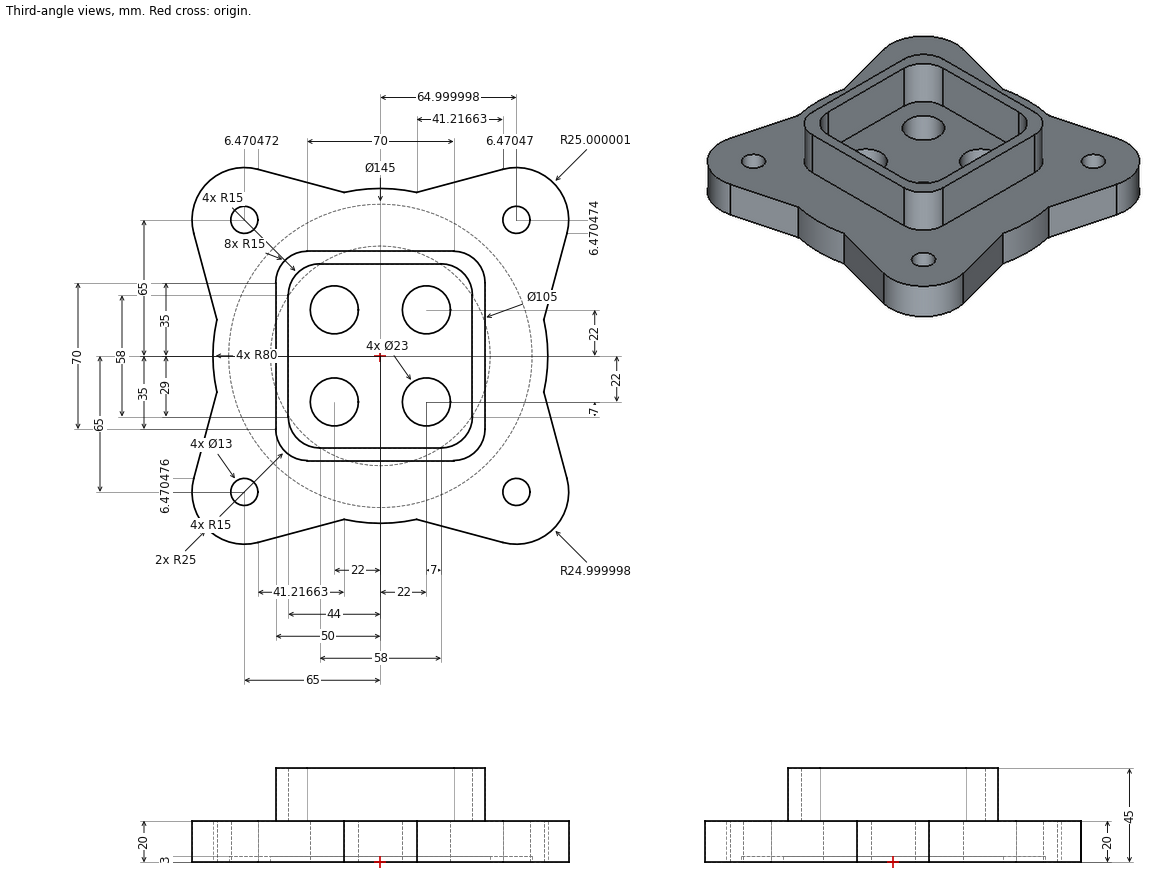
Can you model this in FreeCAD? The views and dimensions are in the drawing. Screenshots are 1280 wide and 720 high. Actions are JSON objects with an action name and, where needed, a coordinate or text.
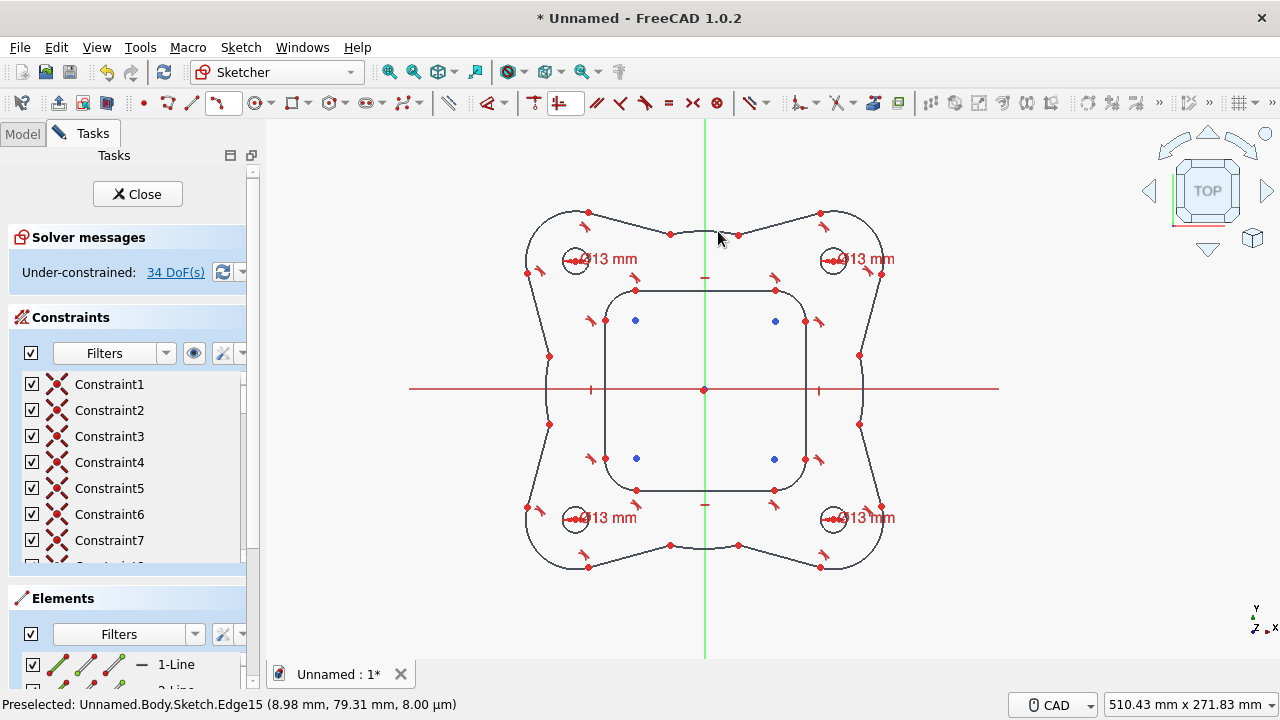
{"action": "scroll", "coordinate": [704, 390], "scroll_direction": "up", "scroll_amount": 6}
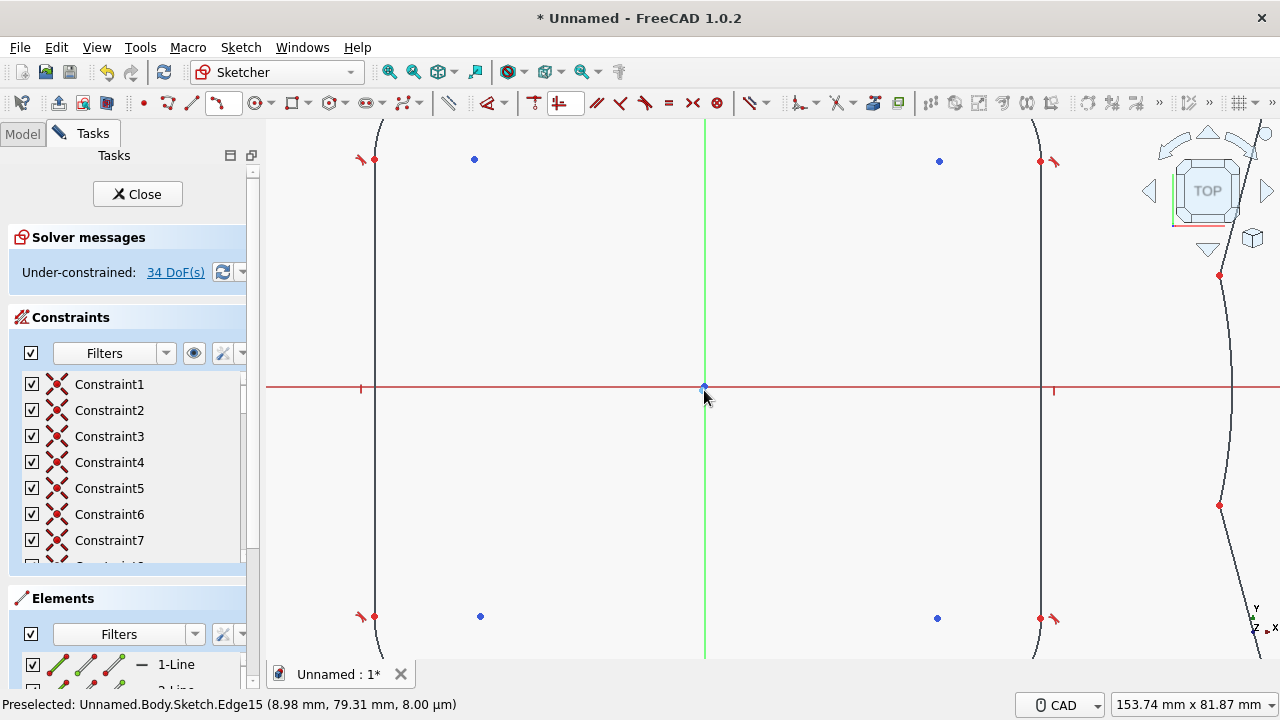
{"action": "left_click_drag", "start_coordinate": [692, 377], "coordinate": [715, 400]}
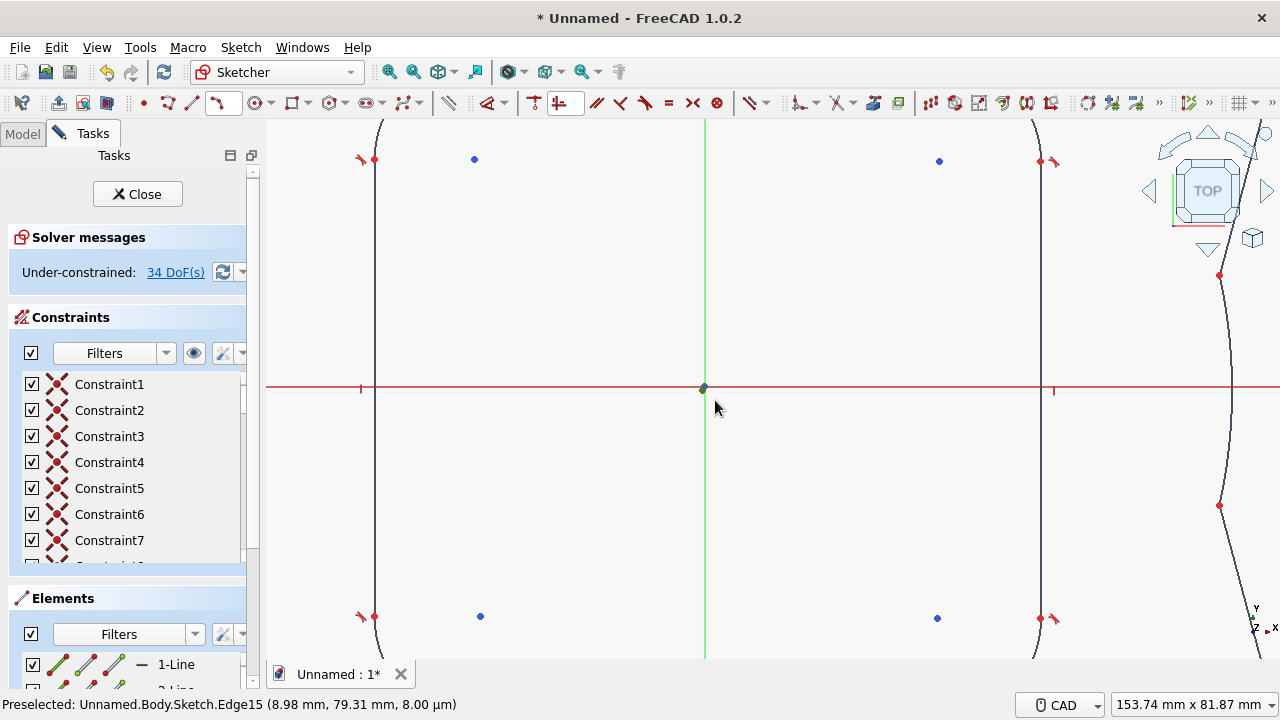
{"action": "left_click", "coordinate": [534, 104]}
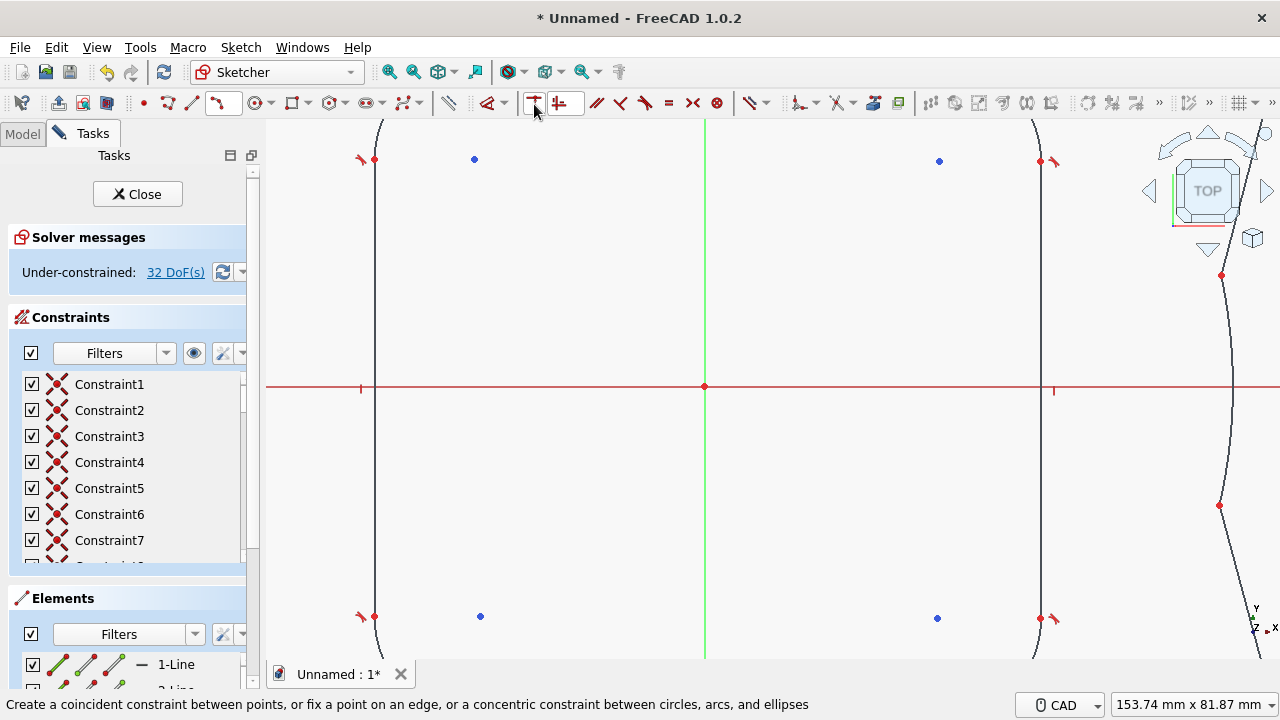
{"action": "scroll", "coordinate": [704, 390], "scroll_direction": "down", "scroll_amount": 6}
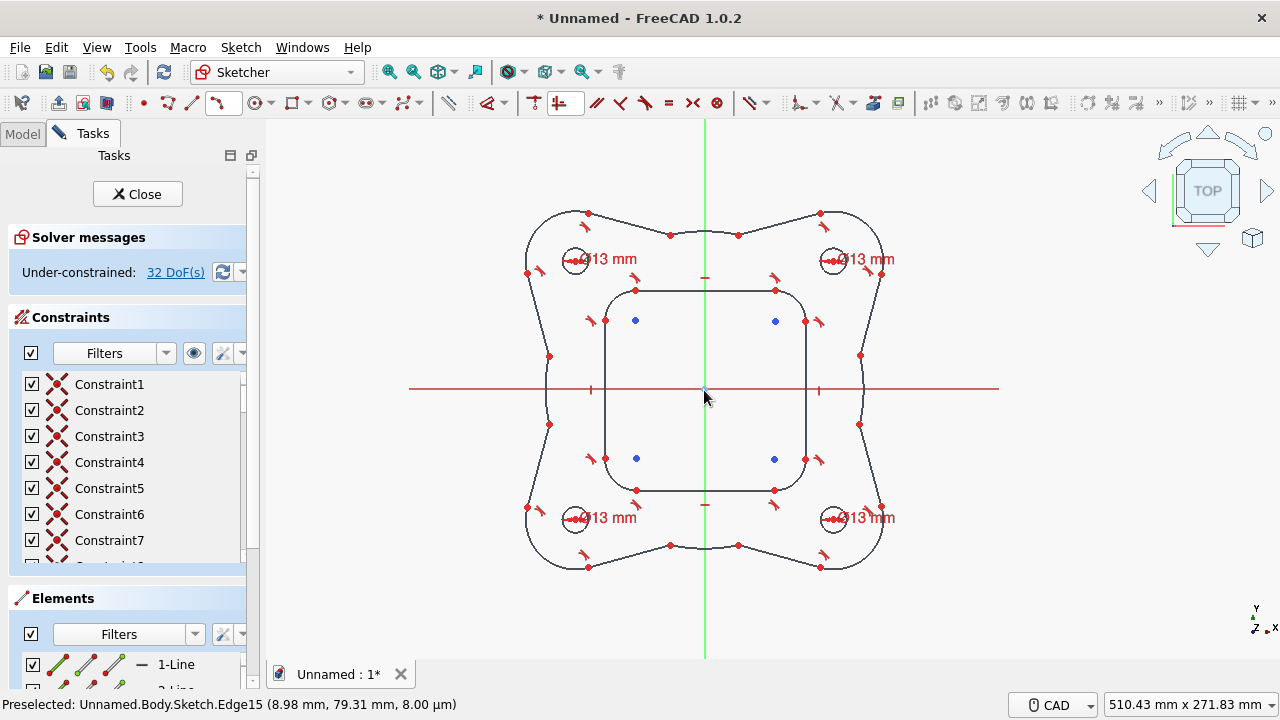
{"action": "left_click", "coordinate": [546, 377]}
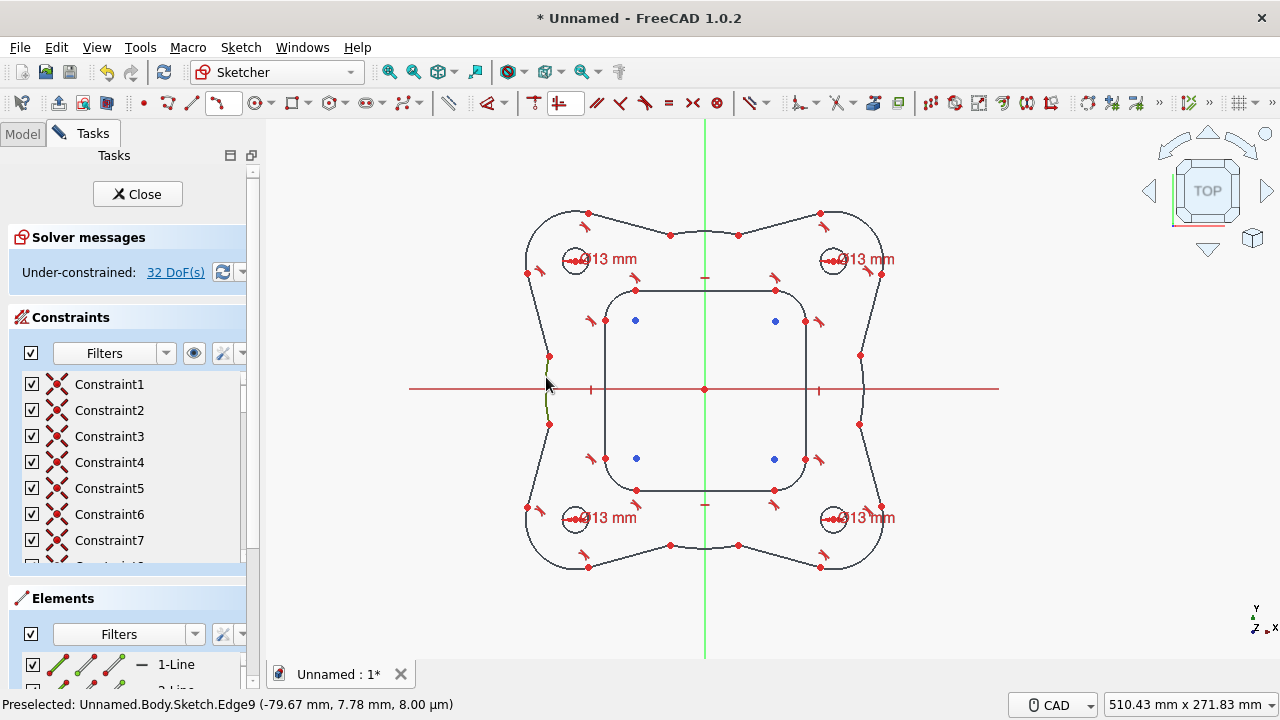
{"action": "left_click", "coordinate": [691, 548]}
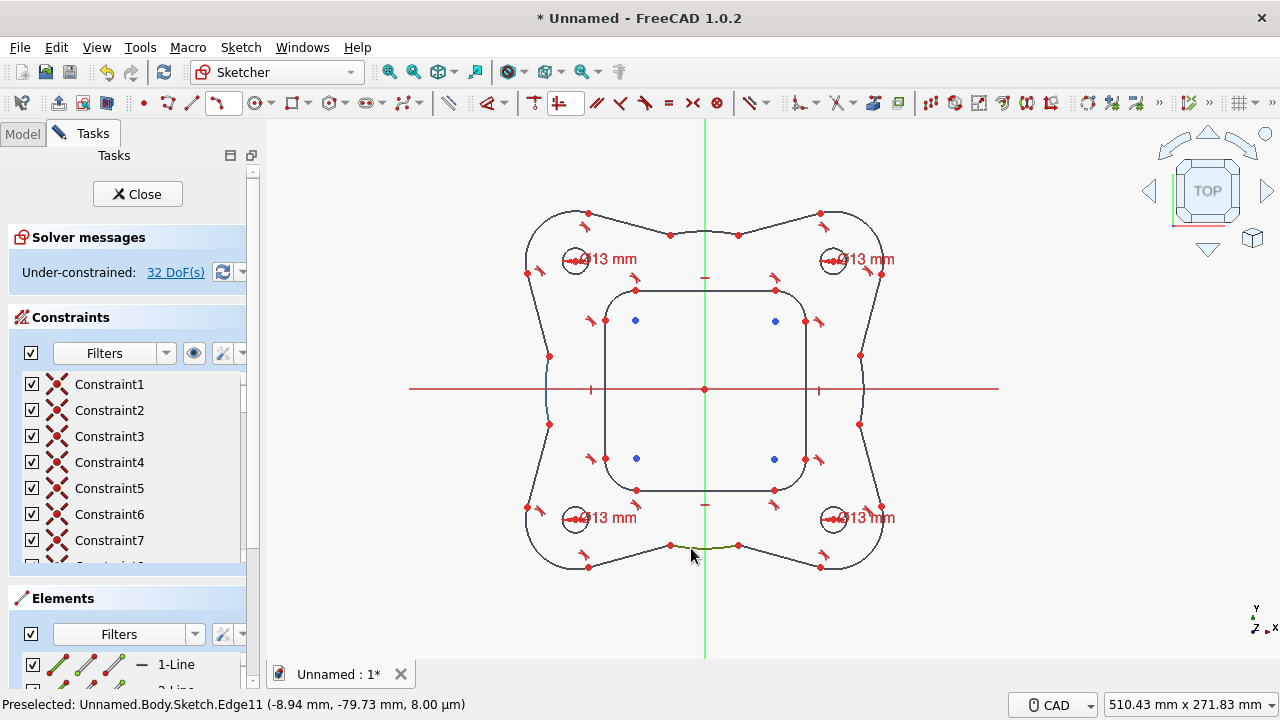
{"action": "left_click", "coordinate": [863, 404]}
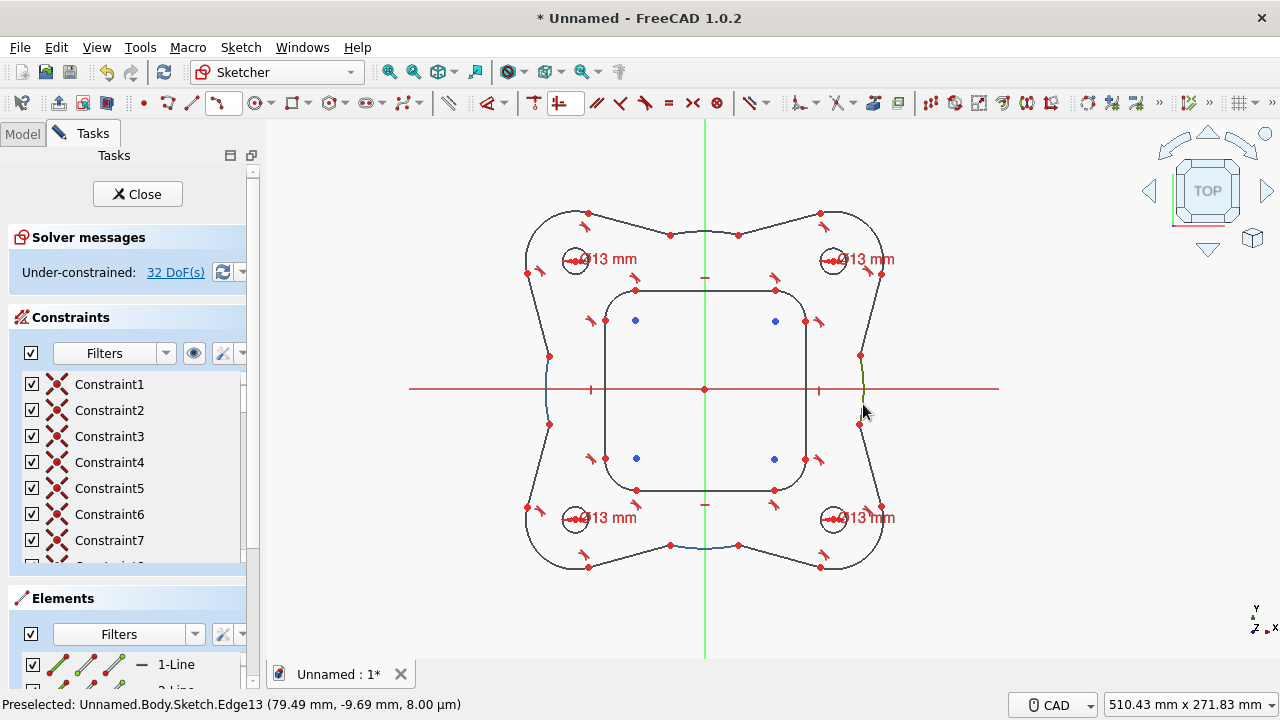
{"action": "left_click", "coordinate": [718, 232]}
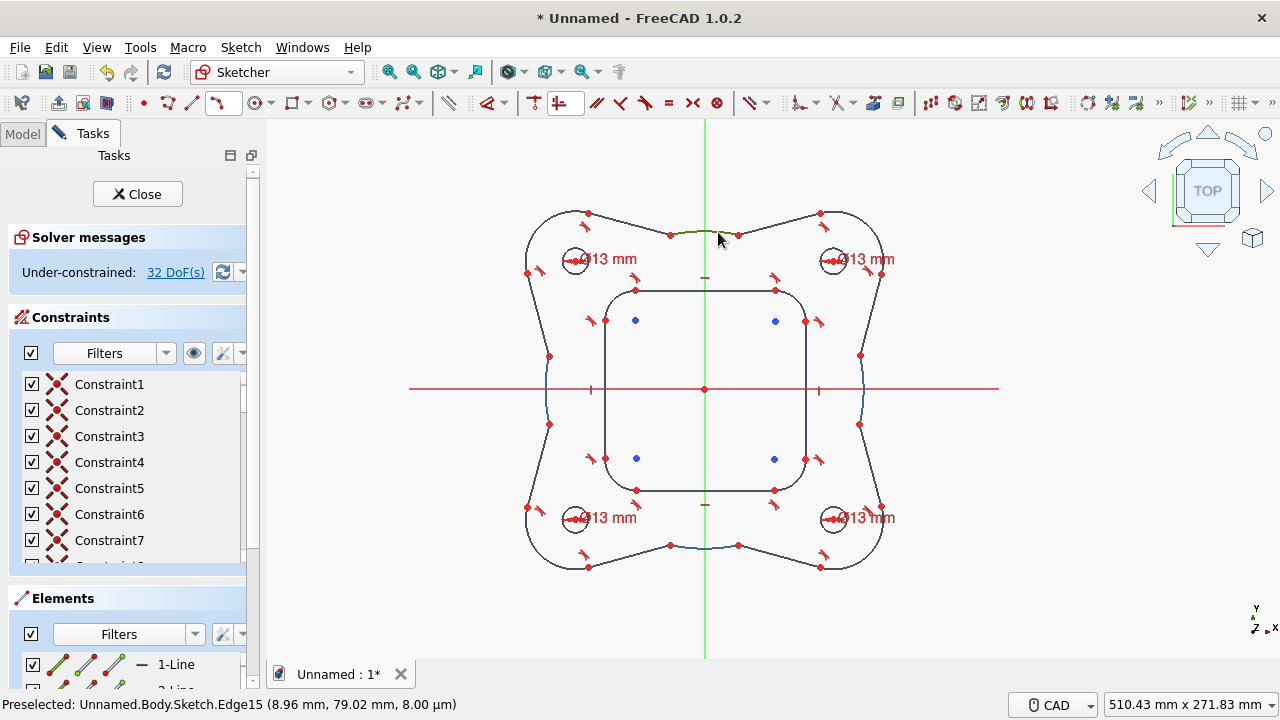
{"action": "key", "text": "e"}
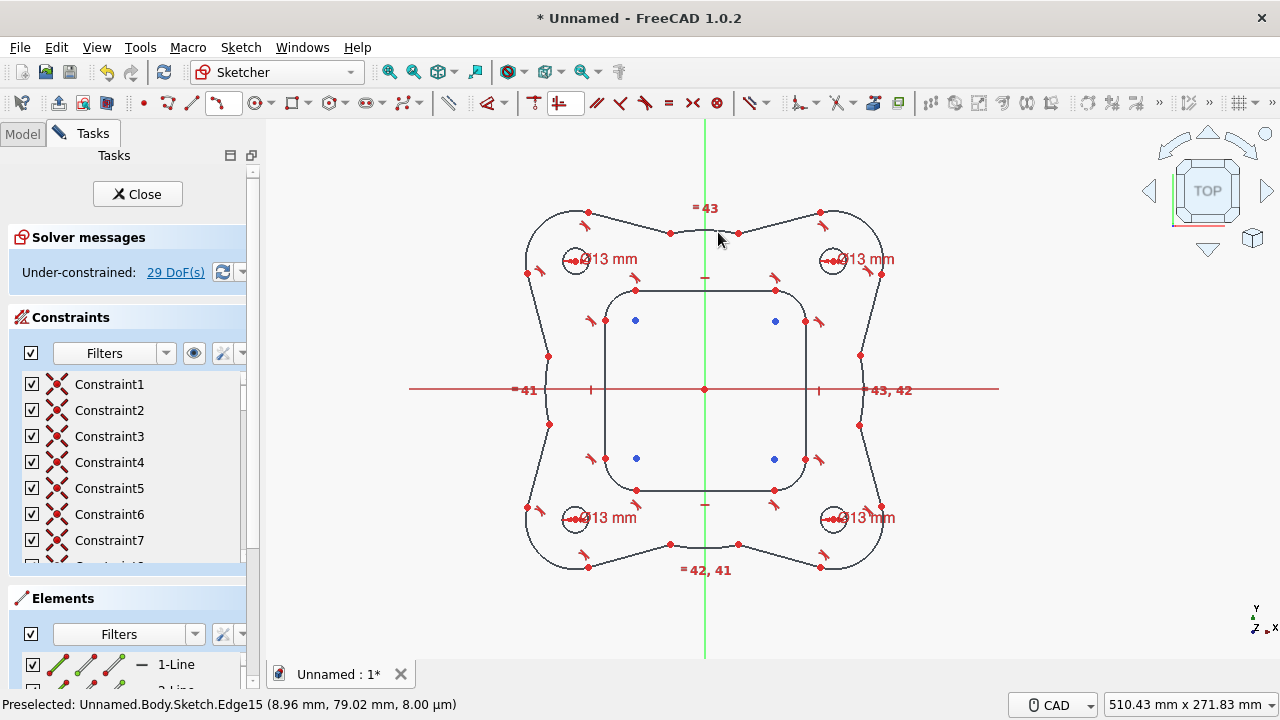
{"action": "left_click", "coordinate": [529, 538]}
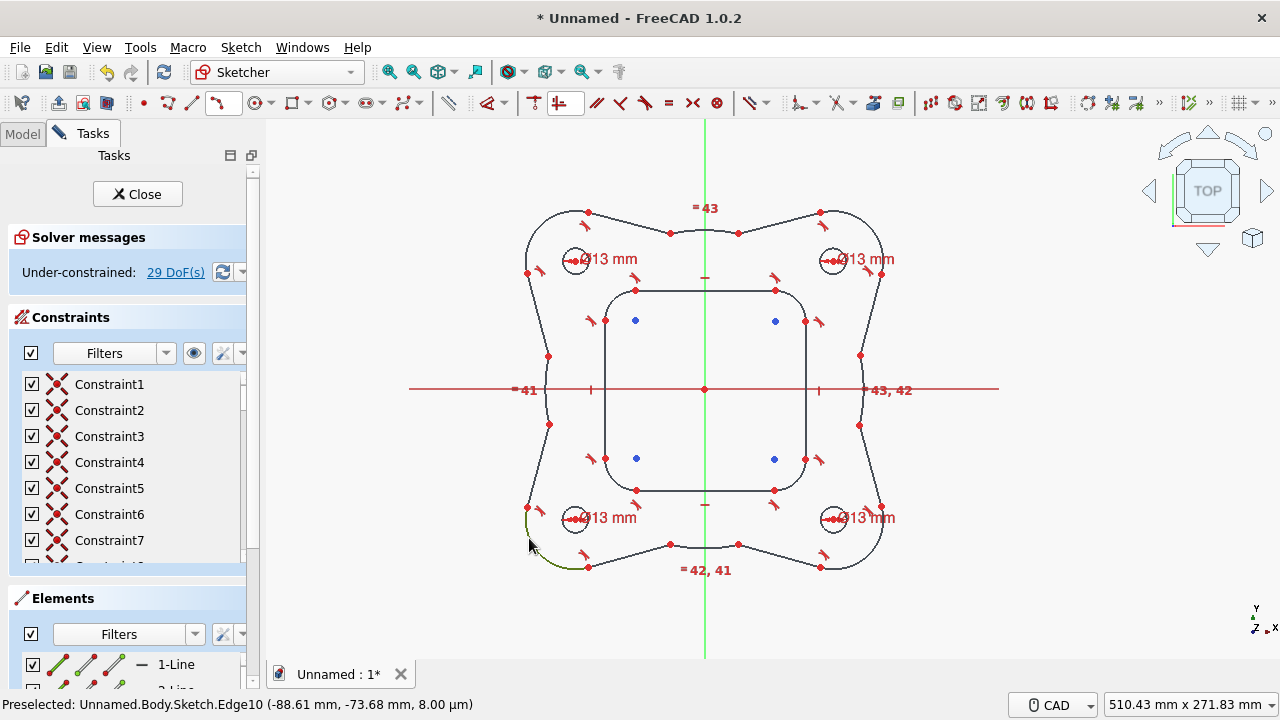
{"action": "left_click", "coordinate": [558, 214]}